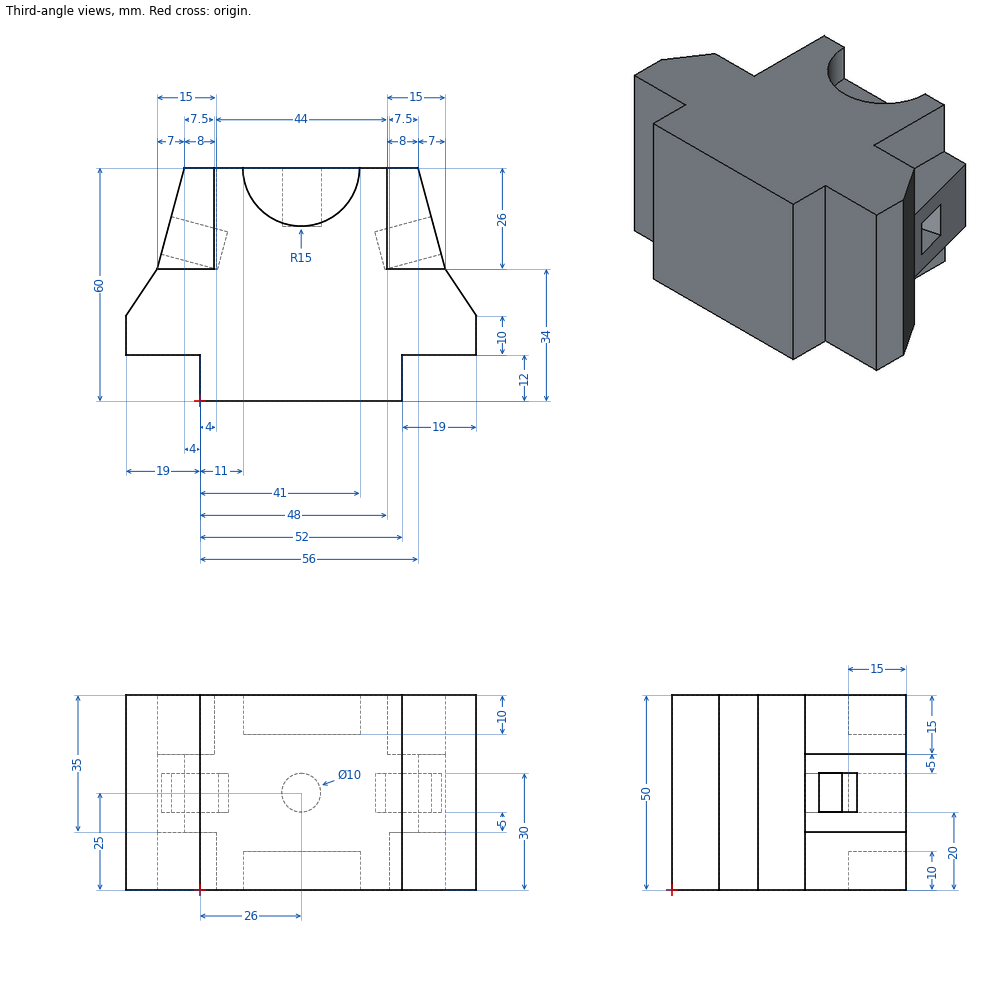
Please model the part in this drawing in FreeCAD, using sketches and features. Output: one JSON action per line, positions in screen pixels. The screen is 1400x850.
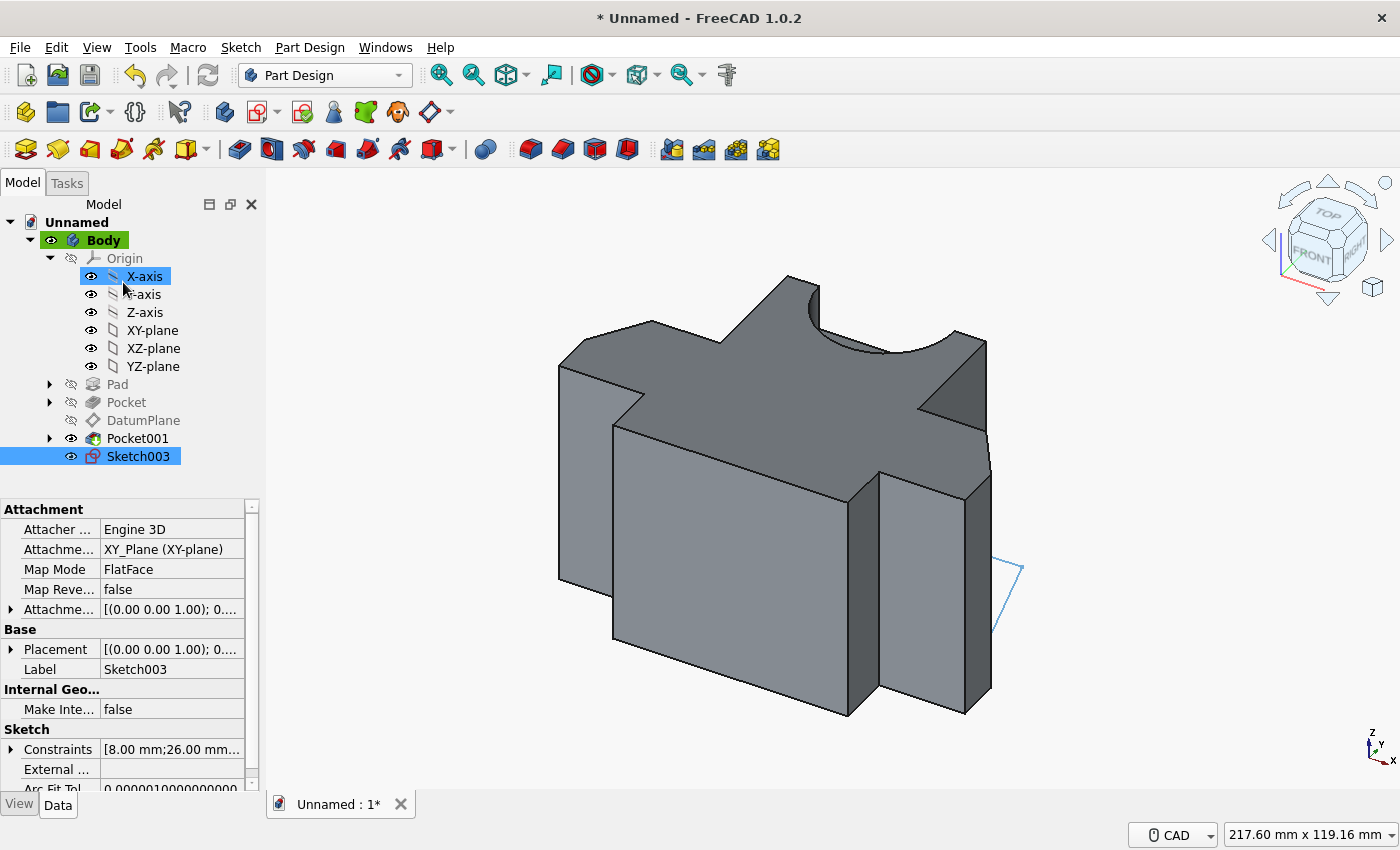
{"action": "left_click", "coordinate": [26, 150]}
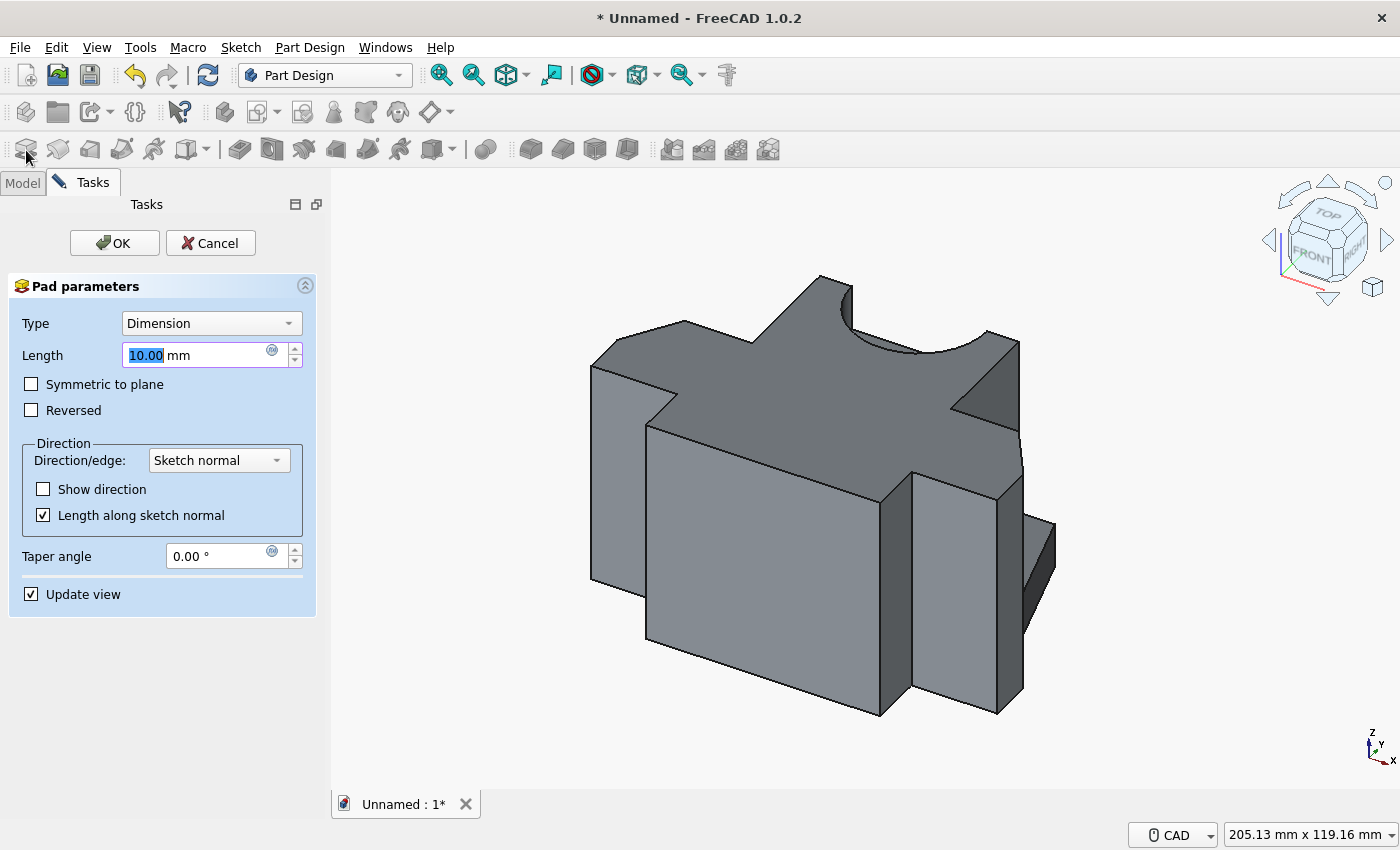
{"action": "type", "text": "30"}
{"action": "key", "text": "Tab"}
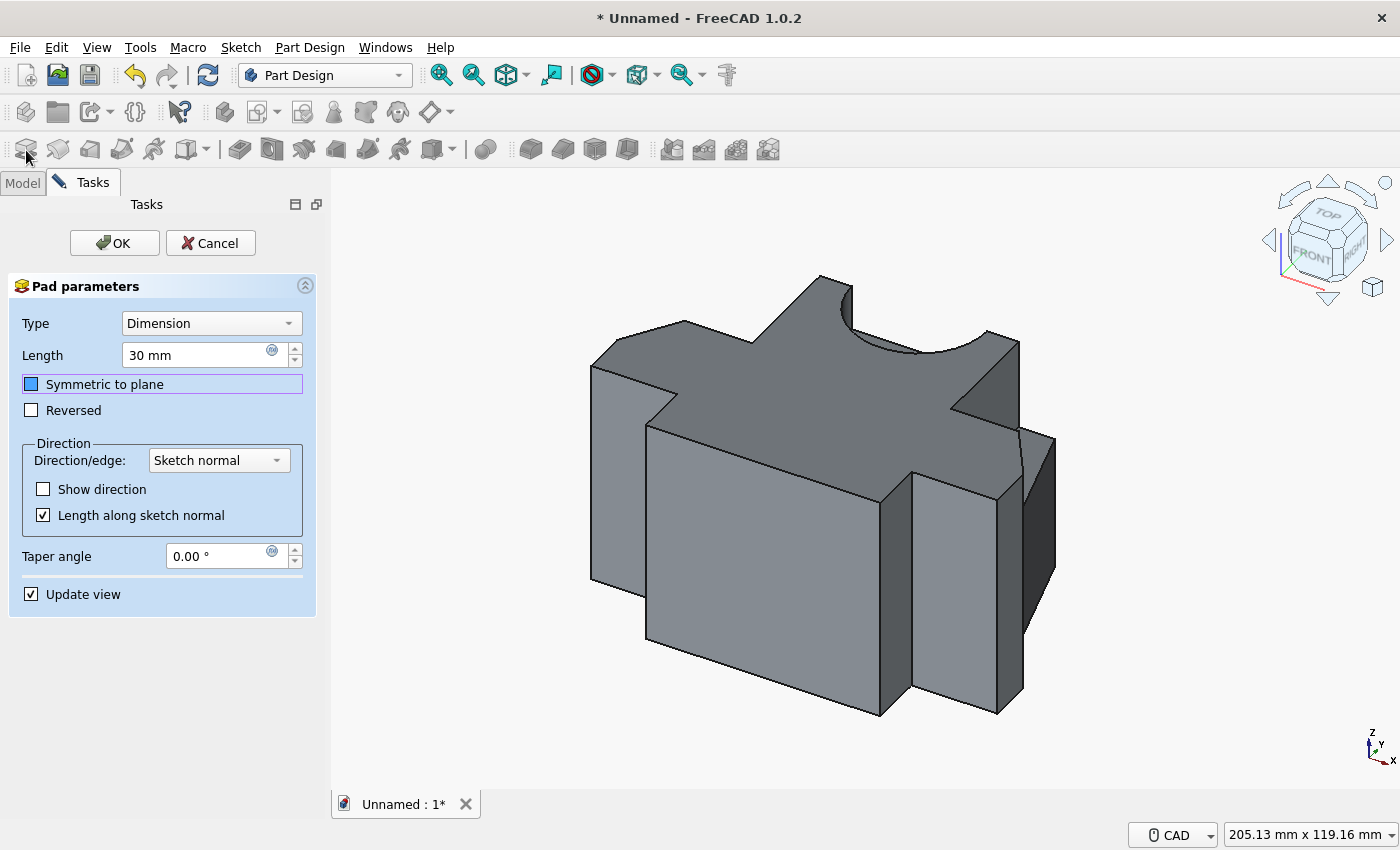
{"action": "left_click", "coordinate": [115, 243]}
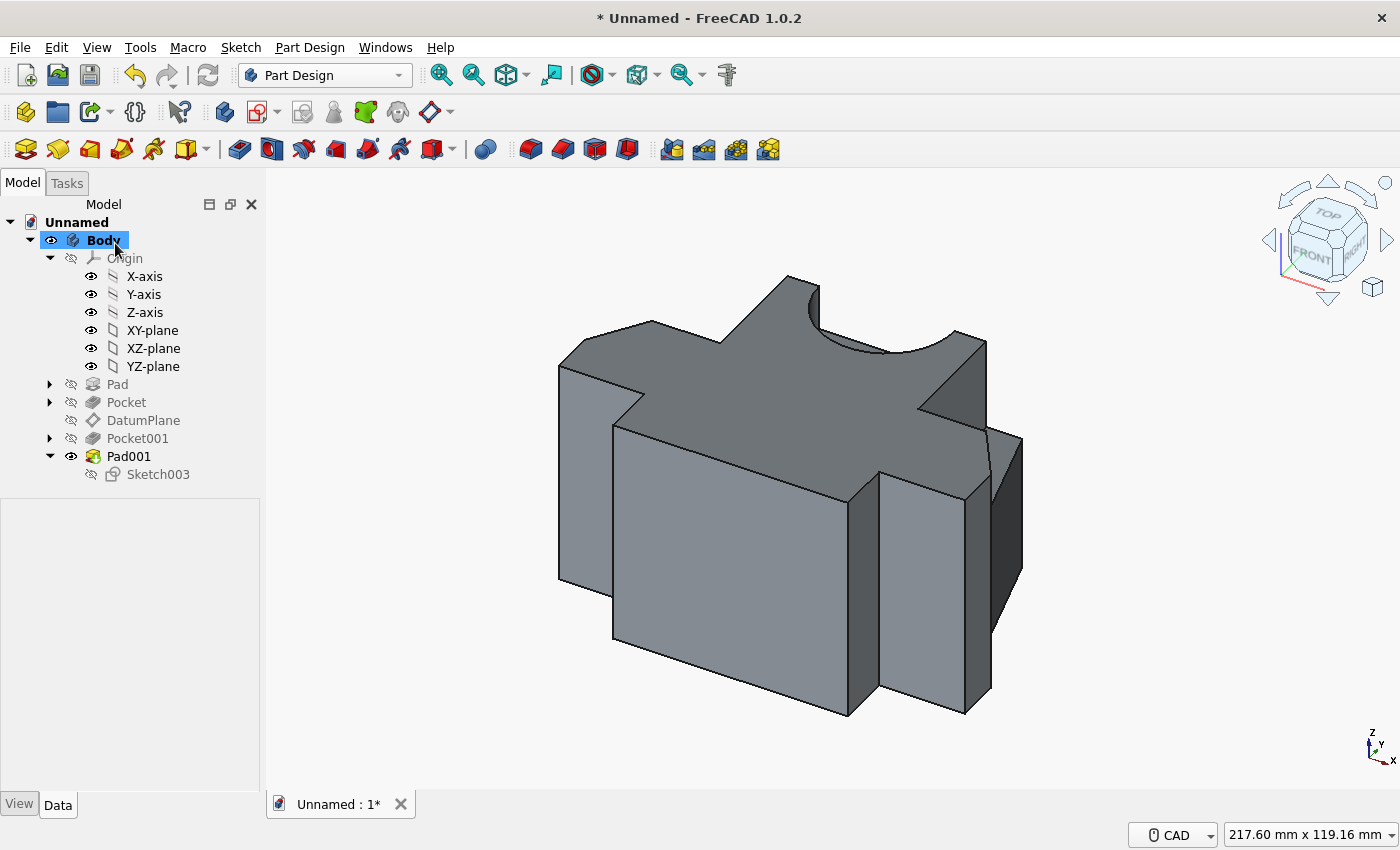
{"action": "left_click", "coordinate": [258, 112]}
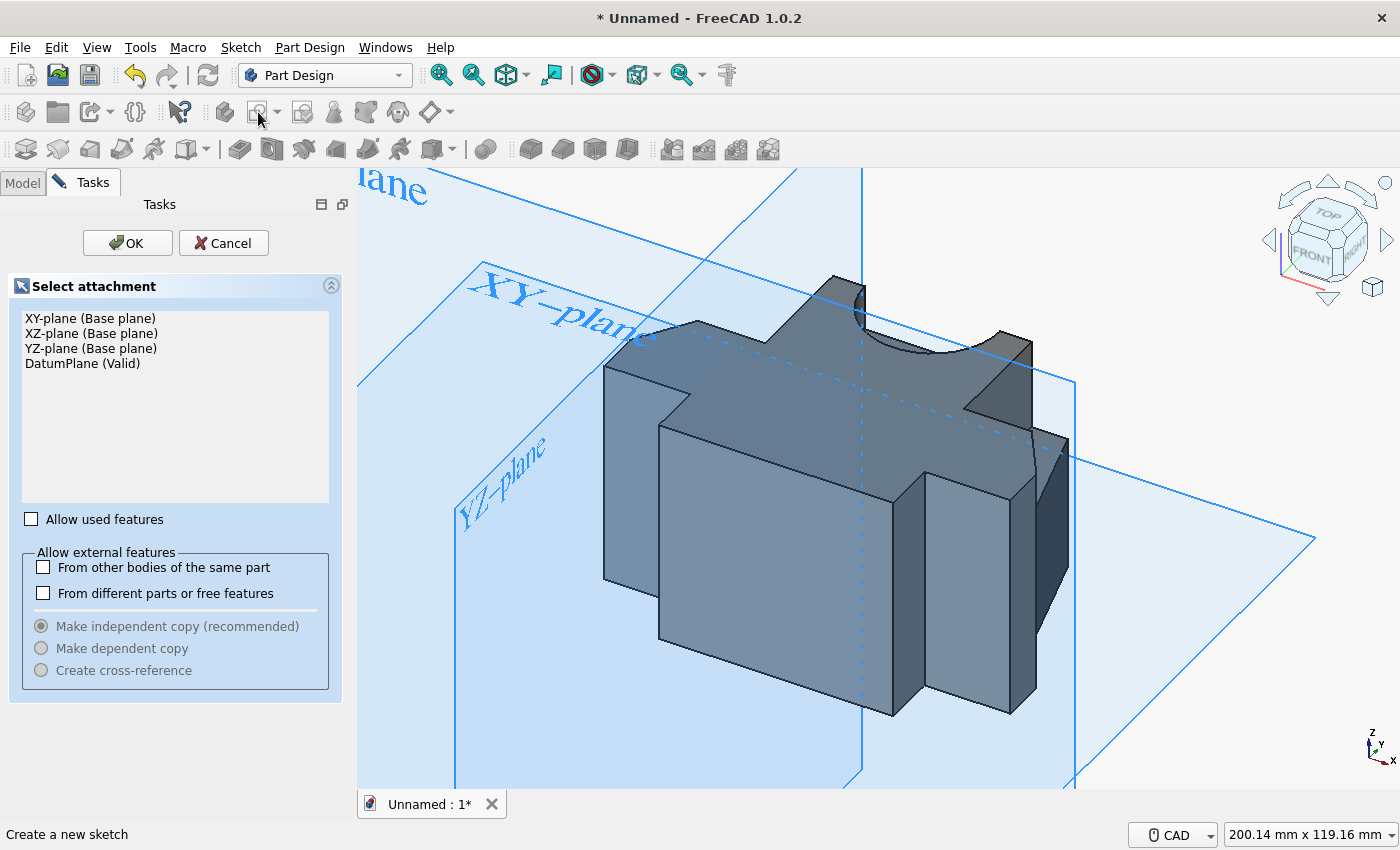
{"action": "left_click", "coordinate": [82, 318]}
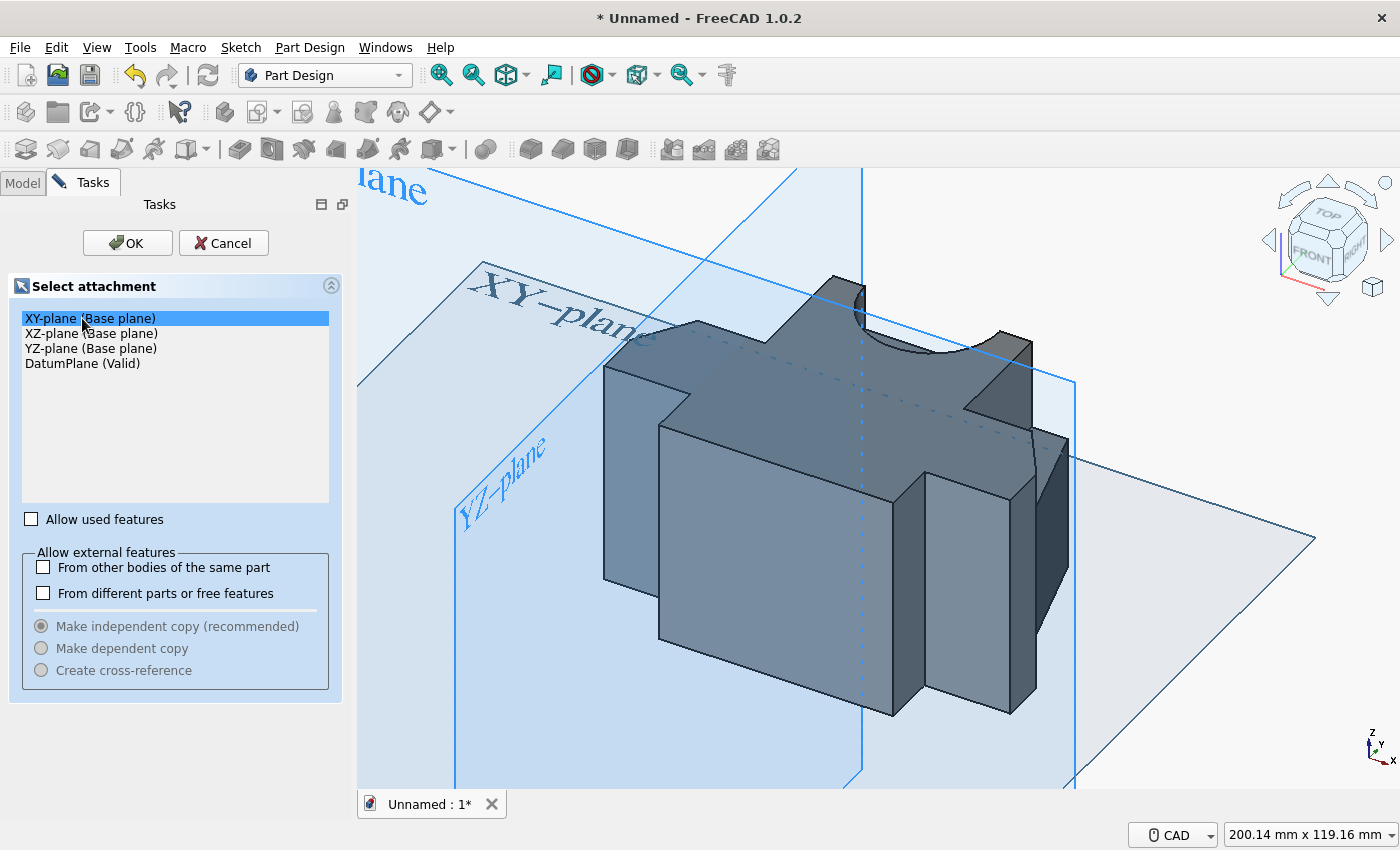
{"action": "left_click", "coordinate": [128, 243]}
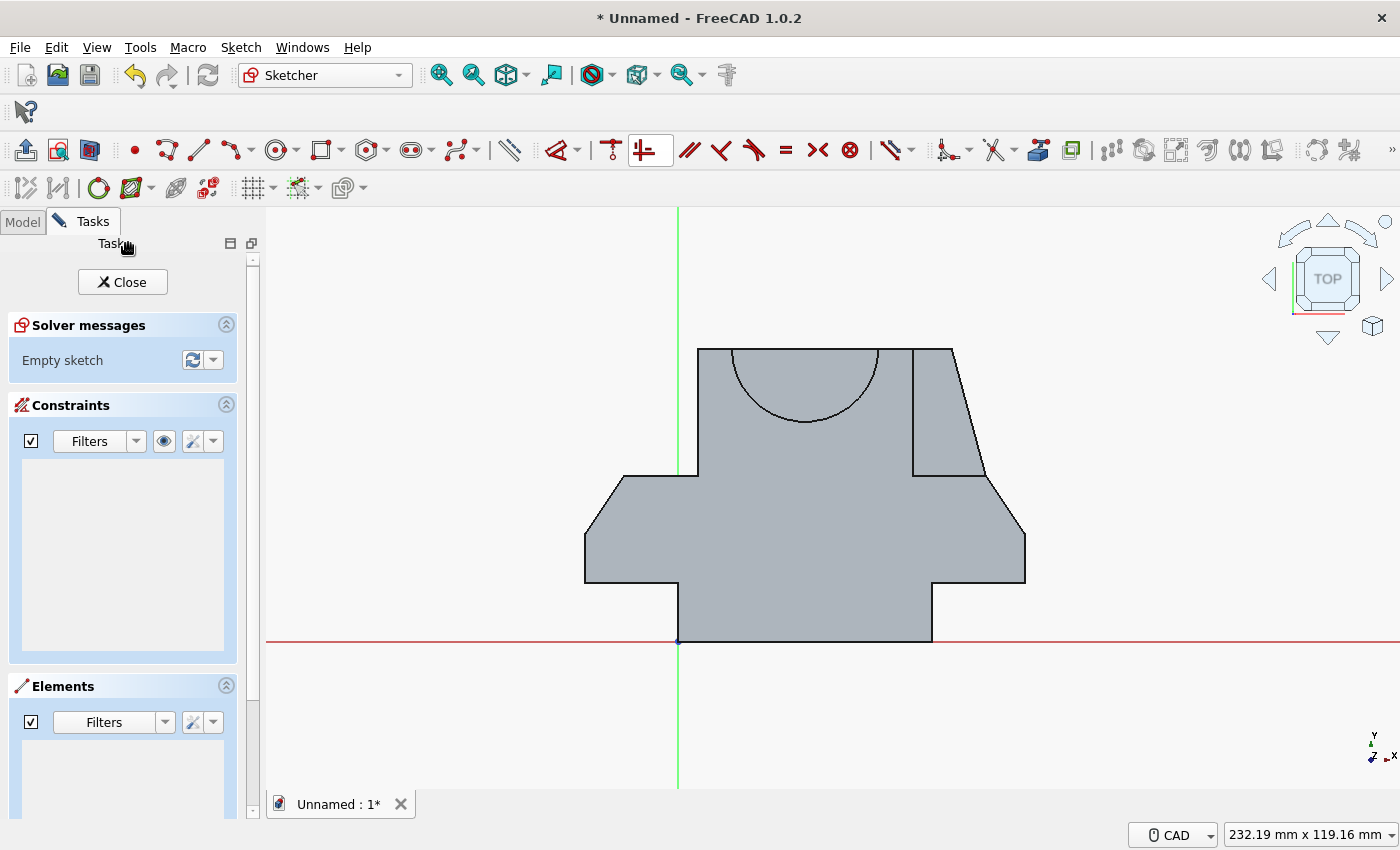
{"action": "left_click", "coordinate": [90, 150]}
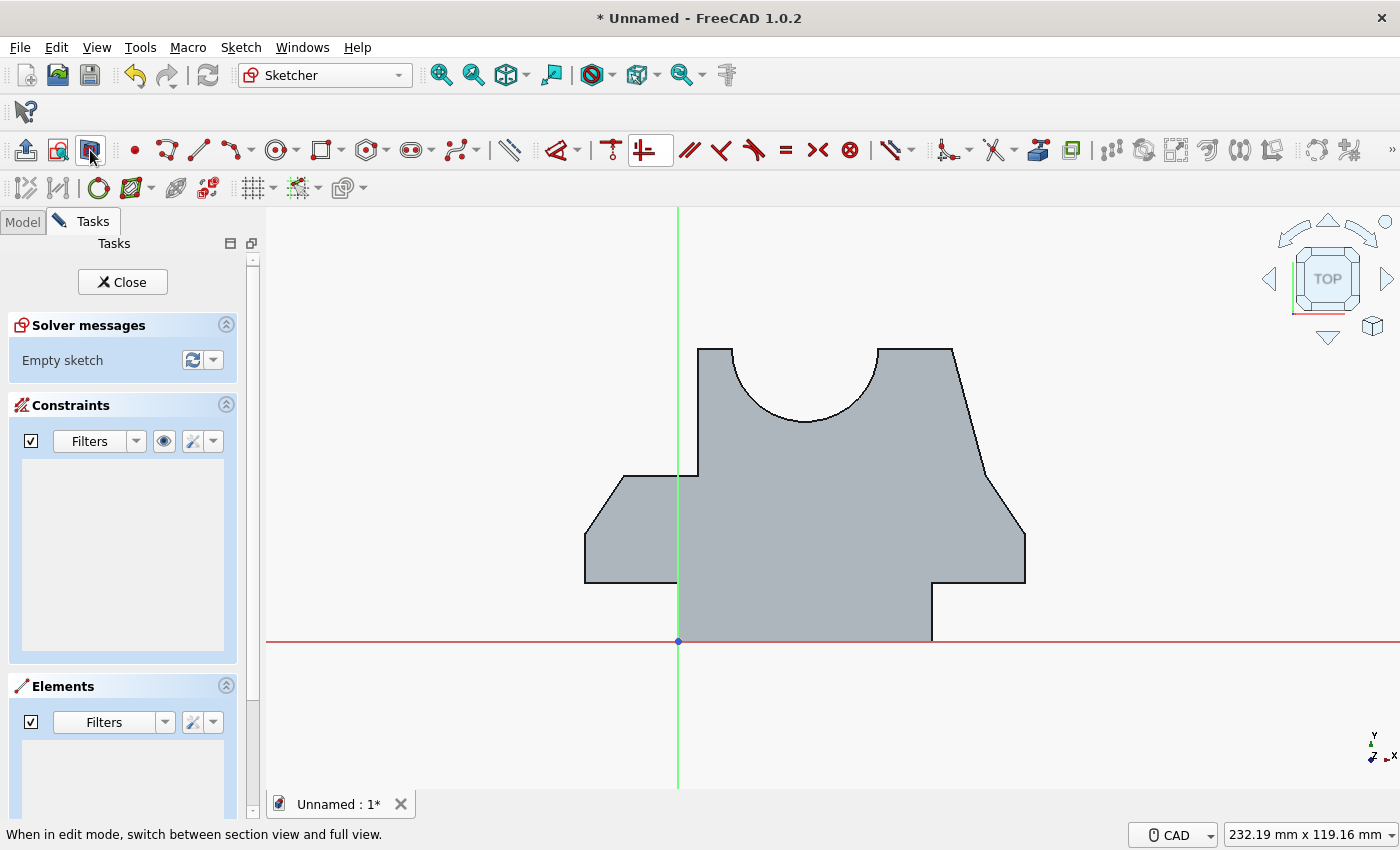
{"action": "left_click", "coordinate": [168, 150]}